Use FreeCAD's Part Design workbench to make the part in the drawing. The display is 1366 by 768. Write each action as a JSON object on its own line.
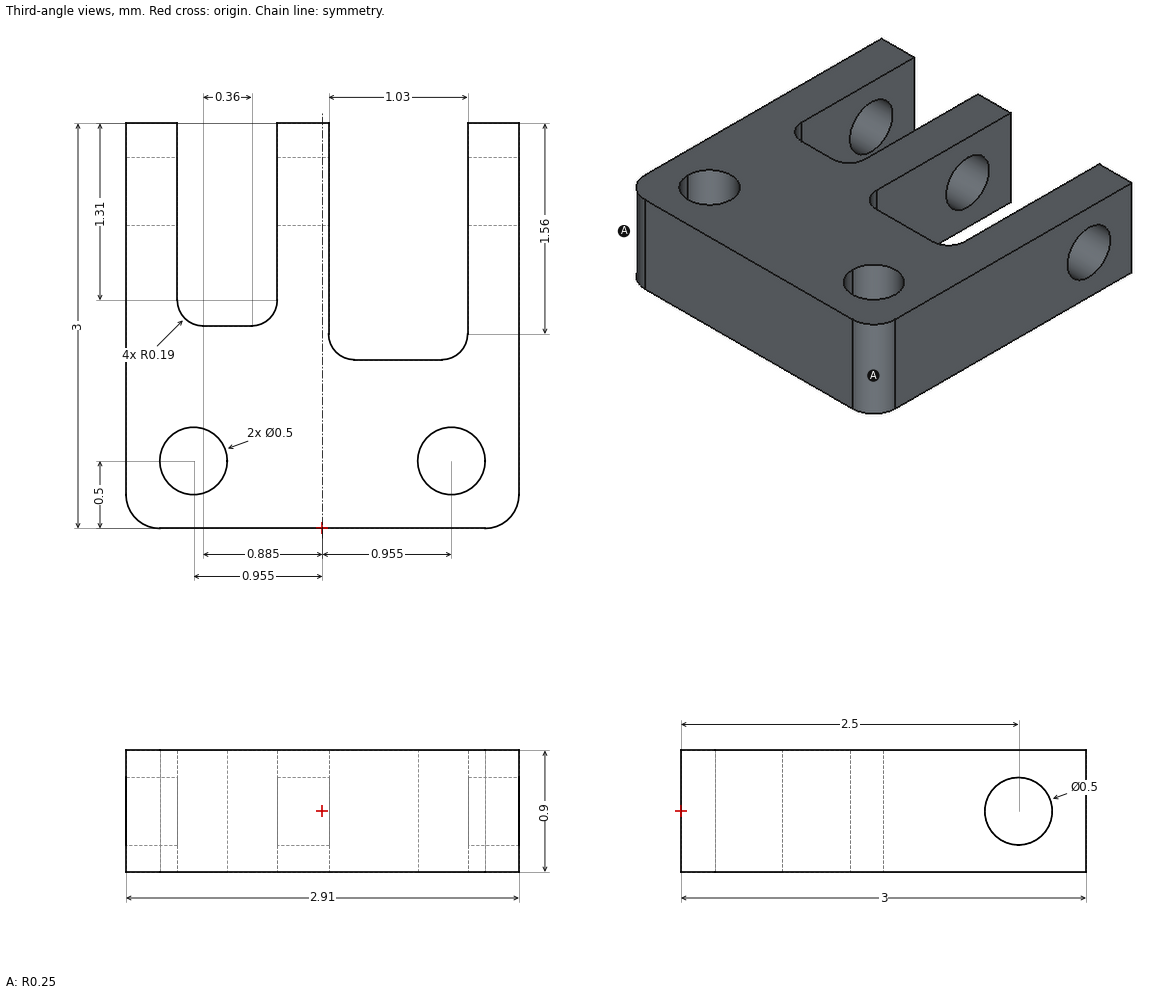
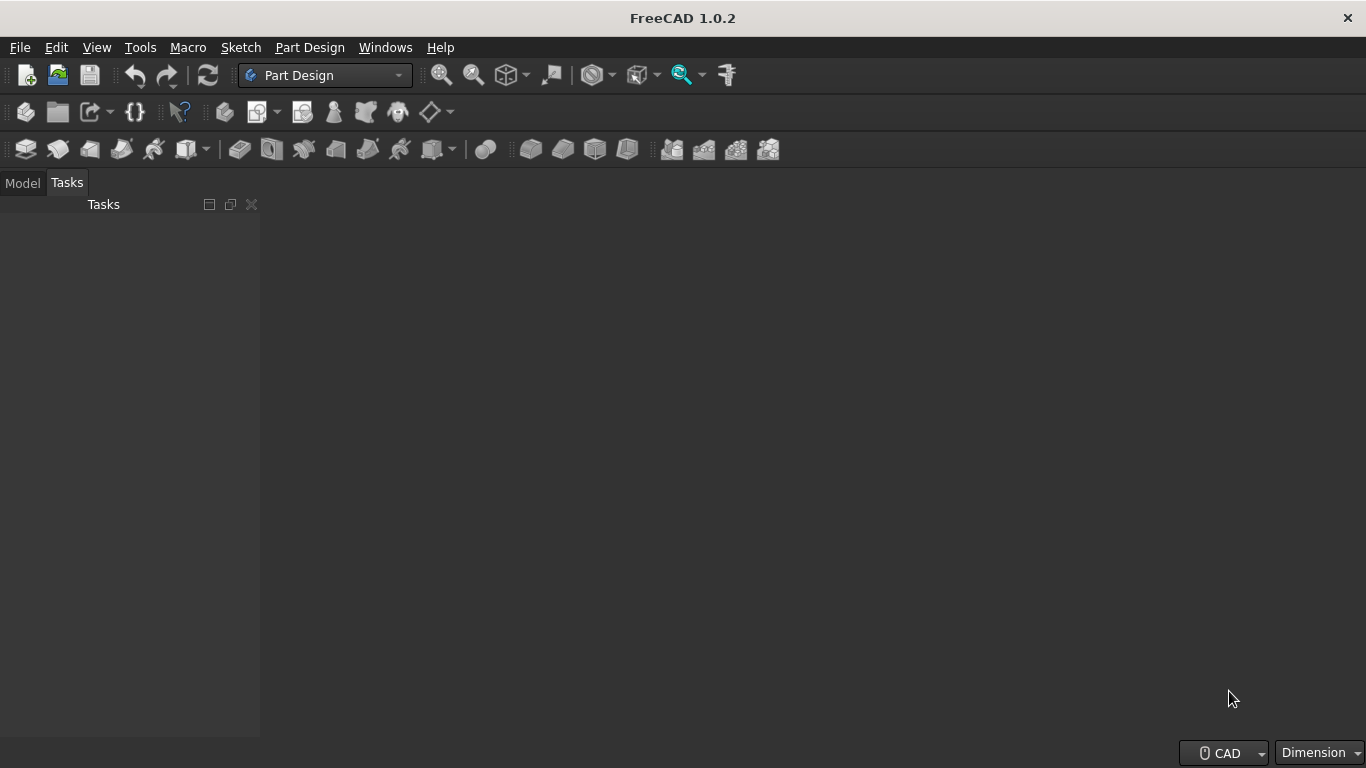
{"action": "key", "text": "ctrl+n"}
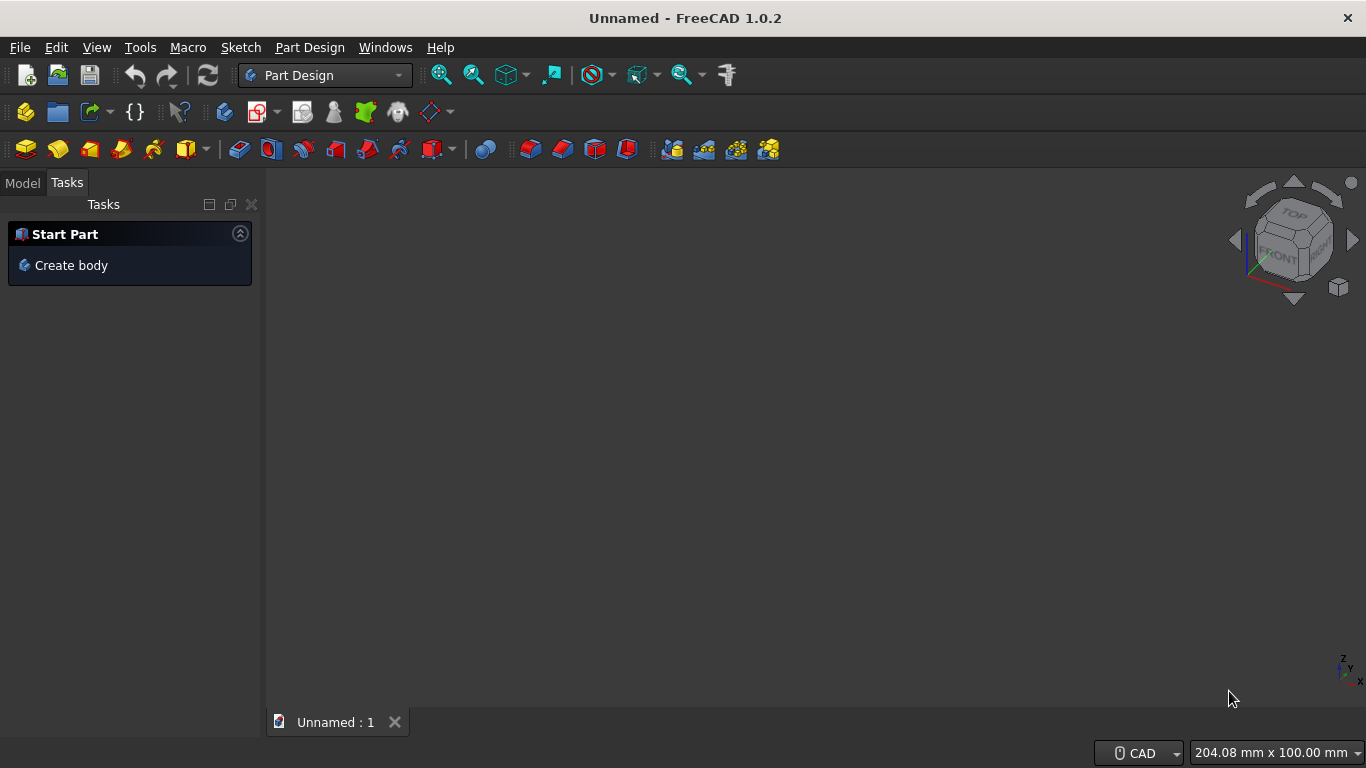
{"action": "left_click", "coordinate": [258, 112]}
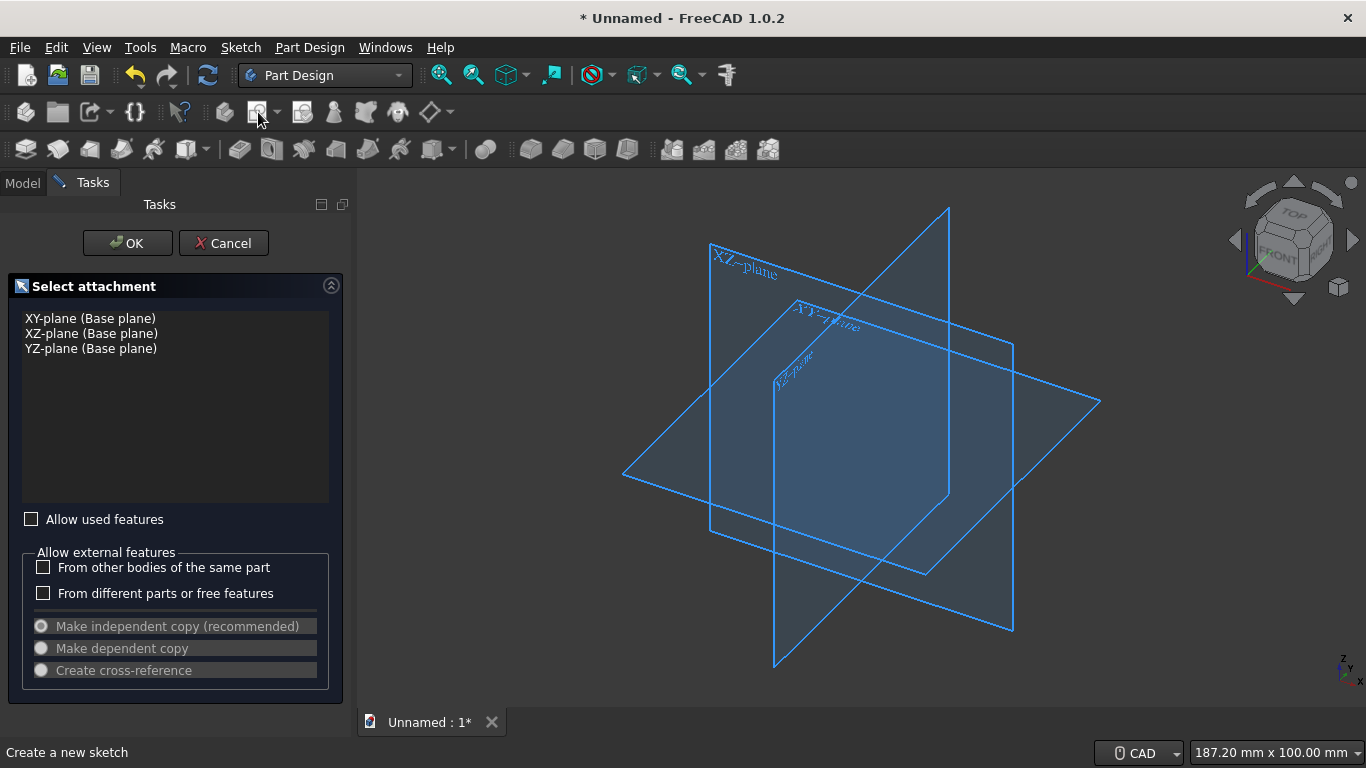
{"action": "left_click", "coordinate": [82, 334]}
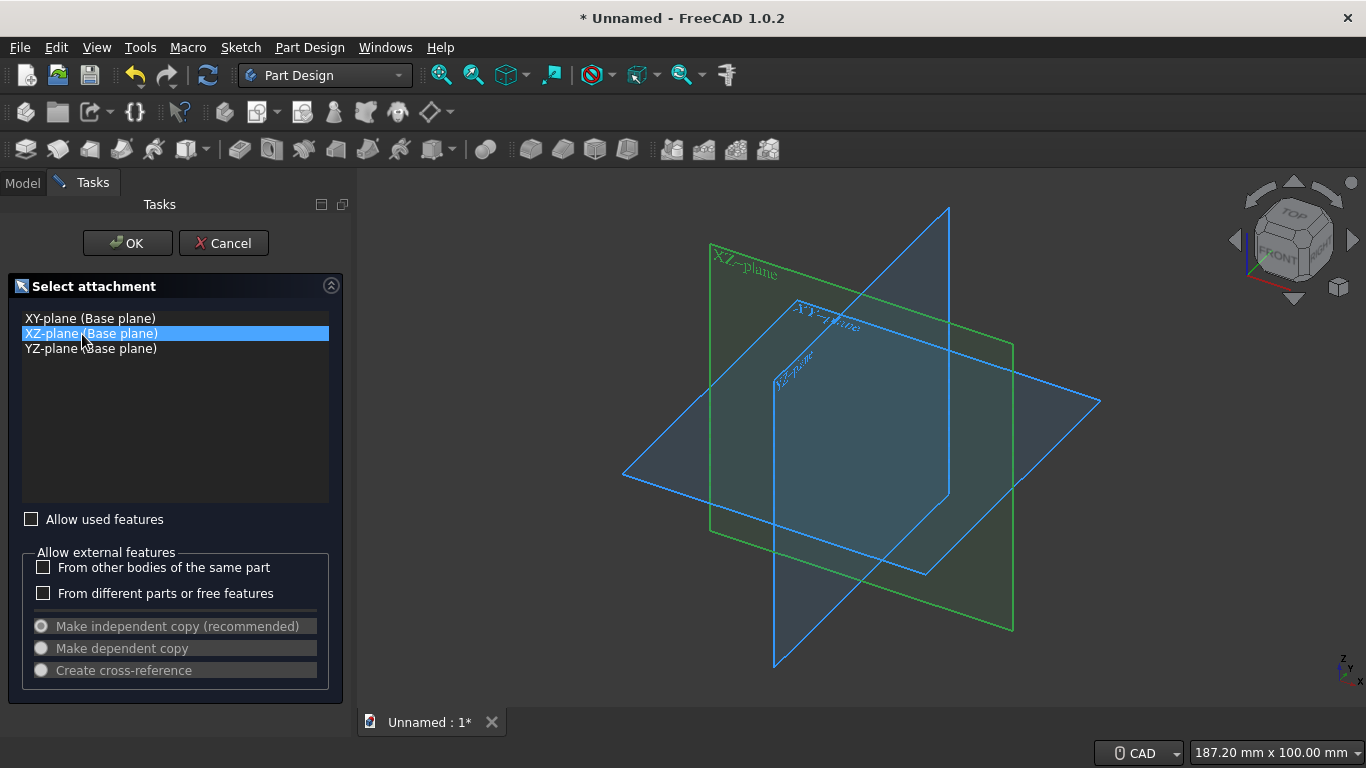
{"action": "left_click", "coordinate": [128, 243]}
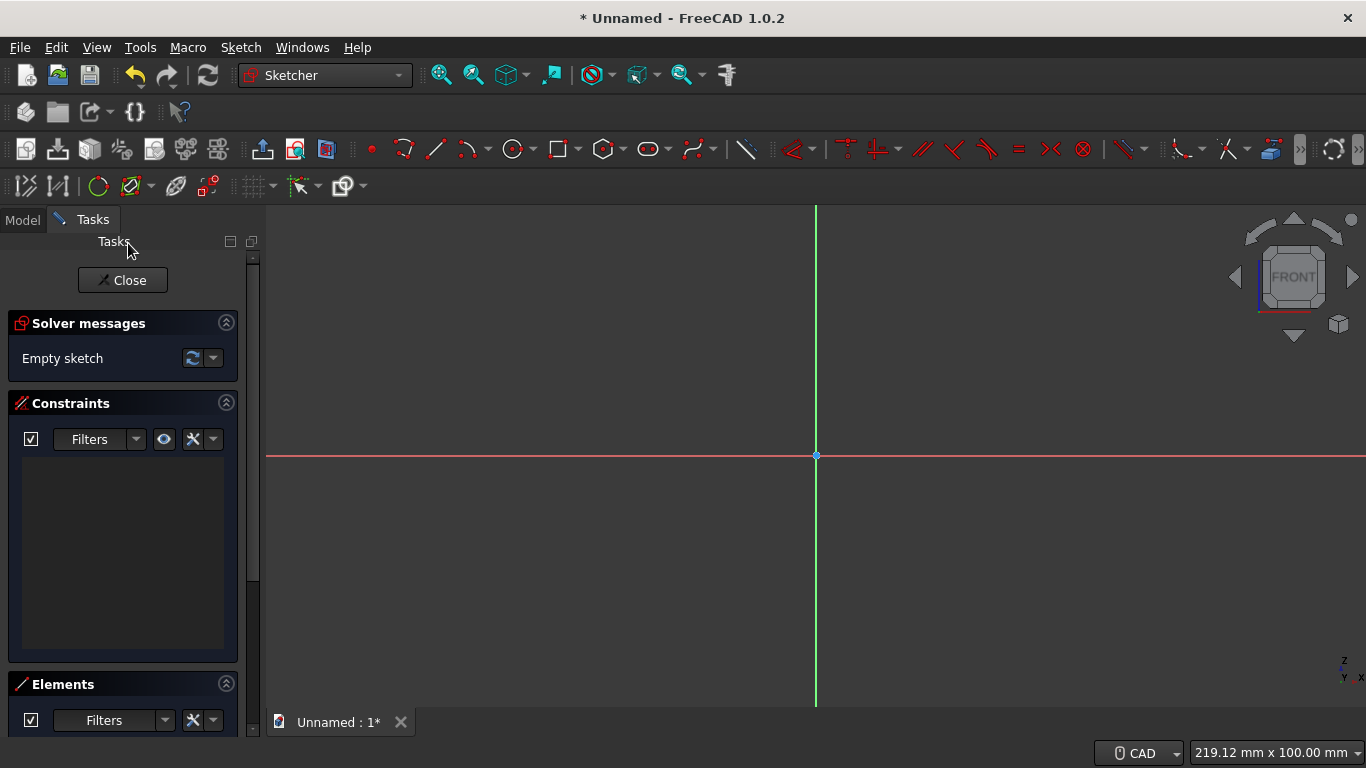
{"action": "scroll", "coordinate": [820, 456], "scroll_direction": "up", "scroll_amount": 15}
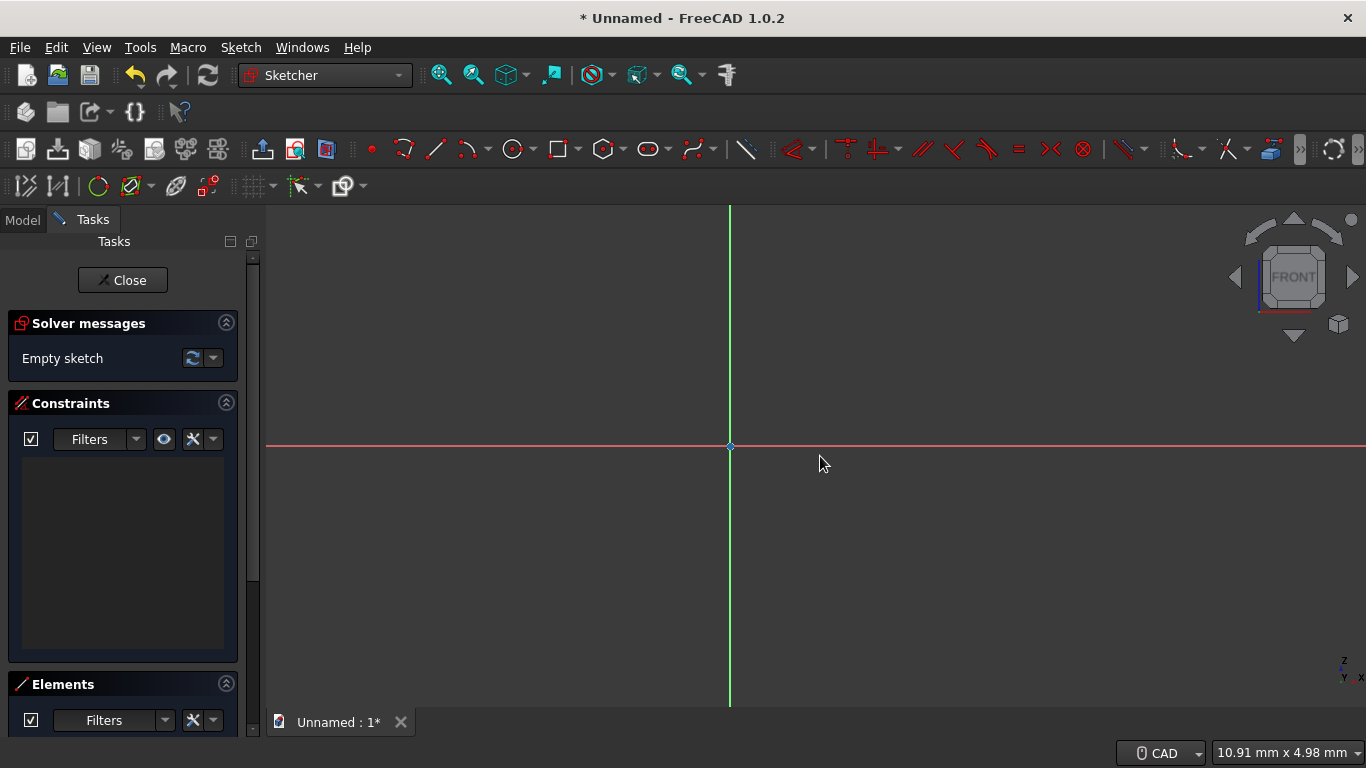
{"action": "scroll", "coordinate": [716, 439], "scroll_direction": "up", "scroll_amount": 4}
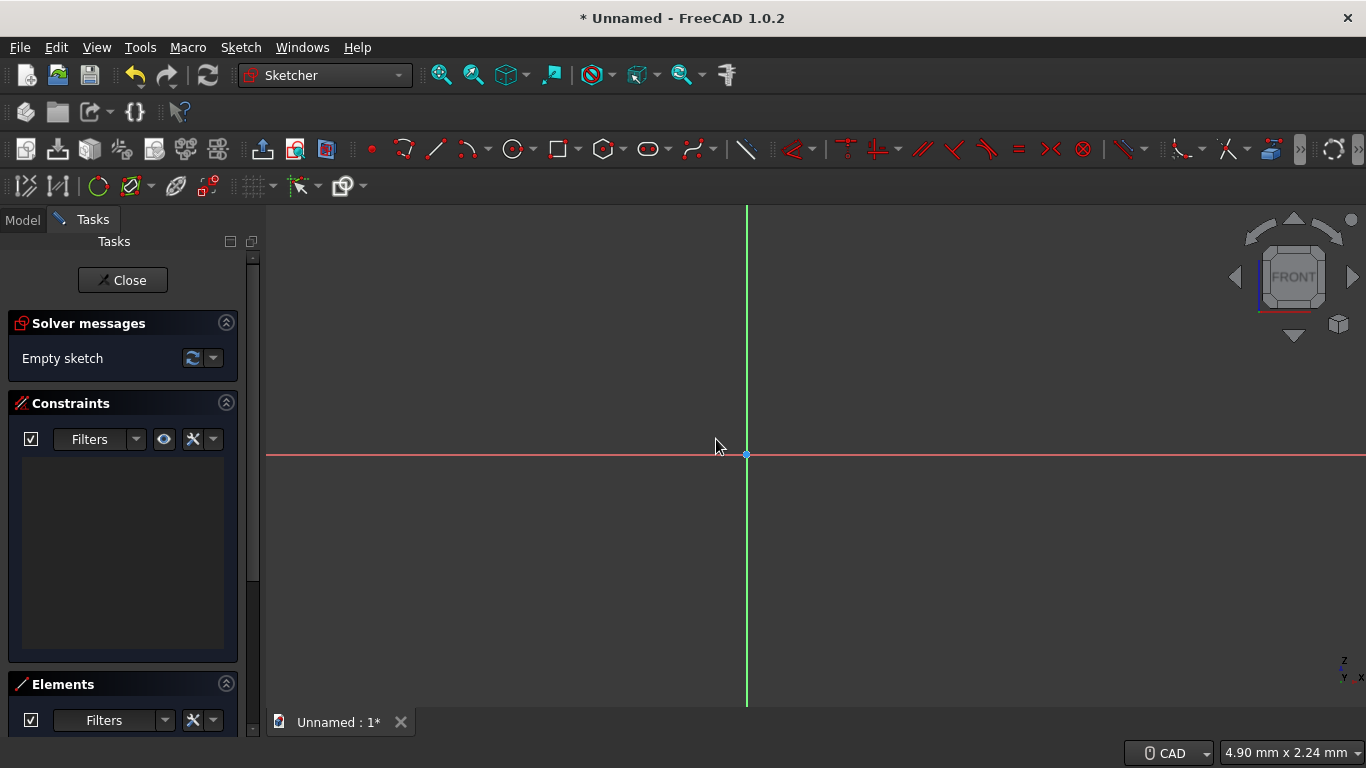
{"action": "key", "text": "g v"}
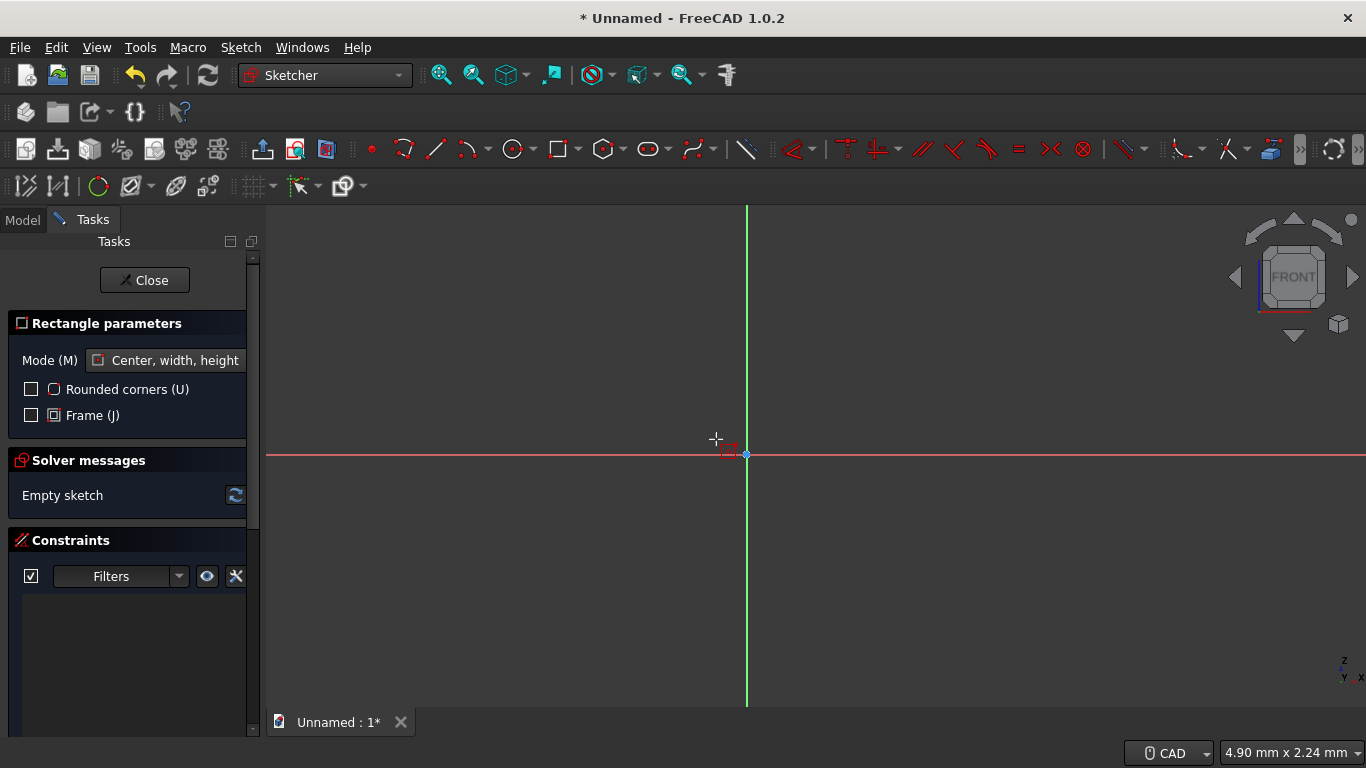
{"action": "left_click", "coordinate": [747, 455]}
{"action": "left_click", "coordinate": [1073, 354]}
{"action": "key", "text": "Escape"}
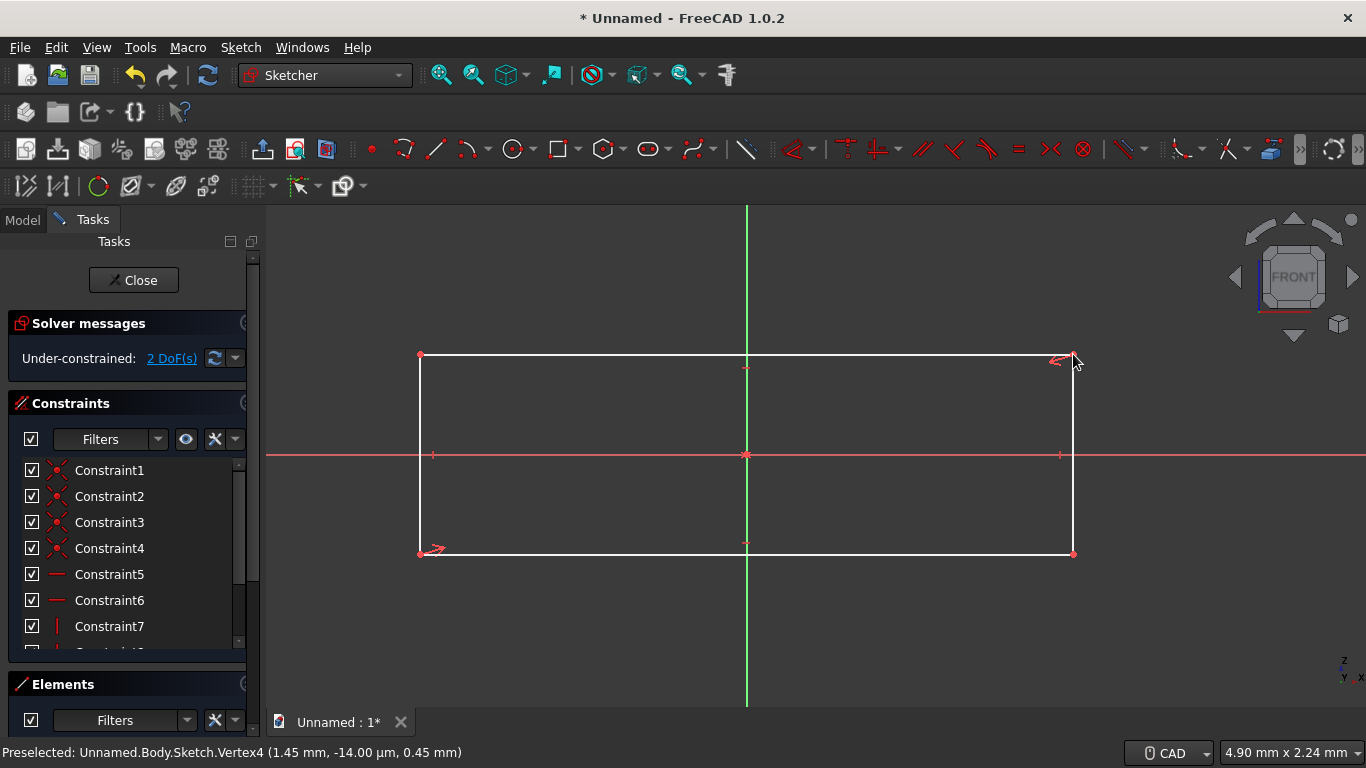
{"action": "key", "text": "d"}